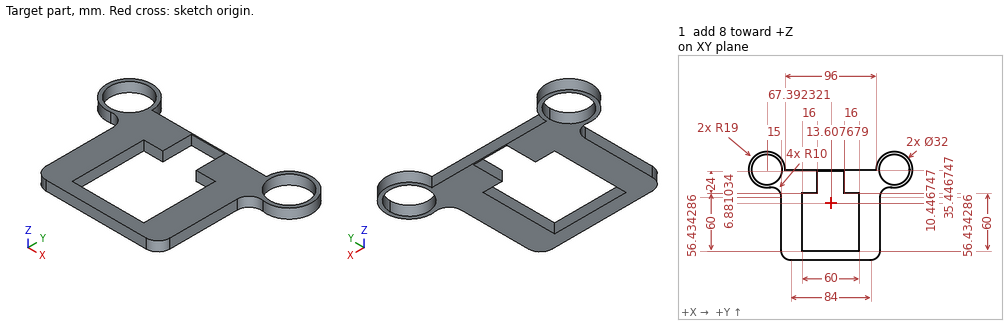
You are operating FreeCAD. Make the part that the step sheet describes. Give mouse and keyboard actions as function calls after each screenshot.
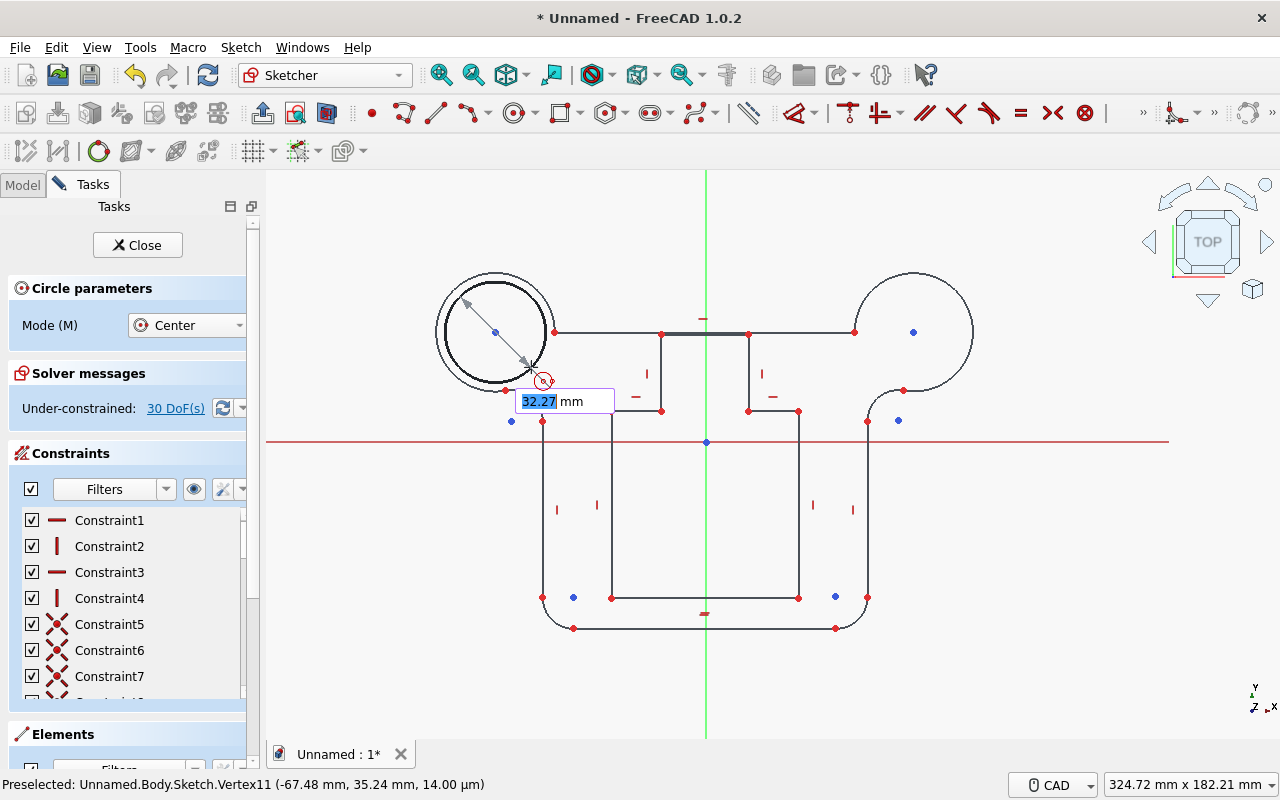
text(32)
key(Return)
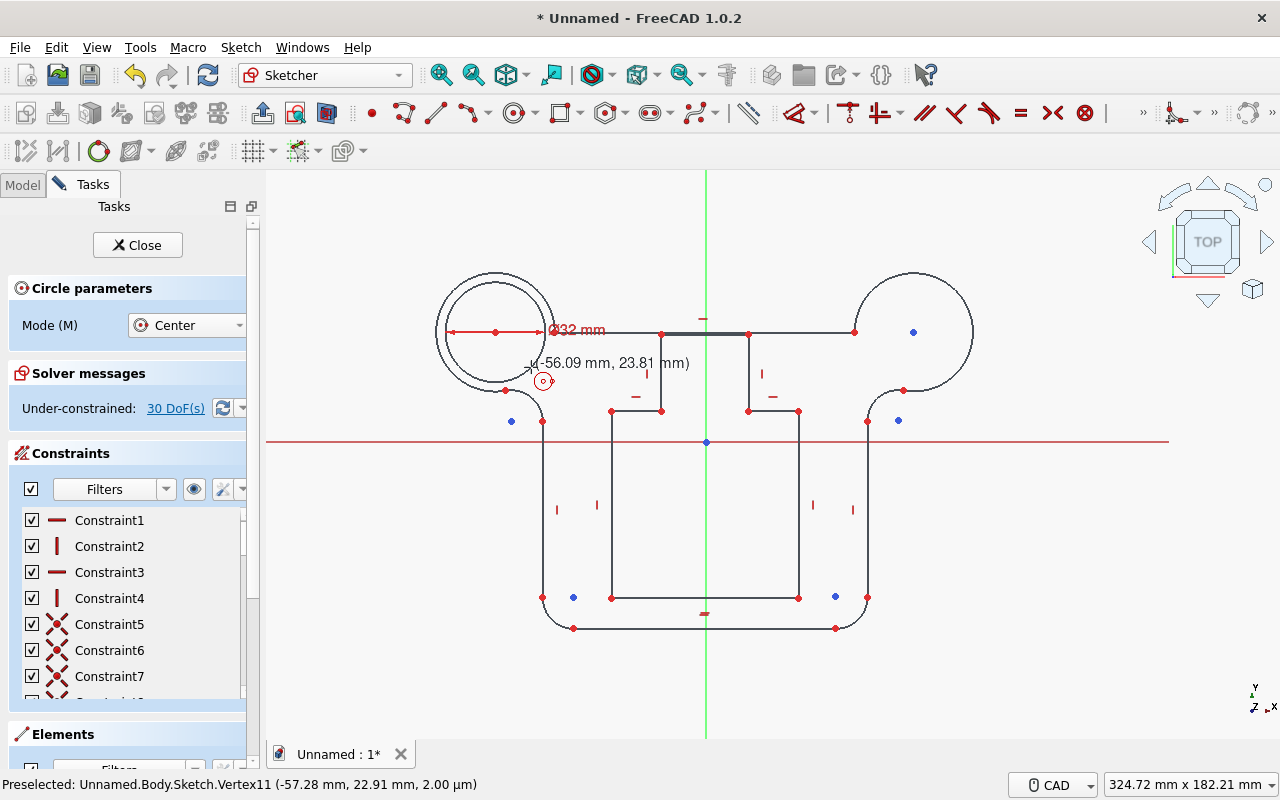
click(914, 332)
move(879, 367)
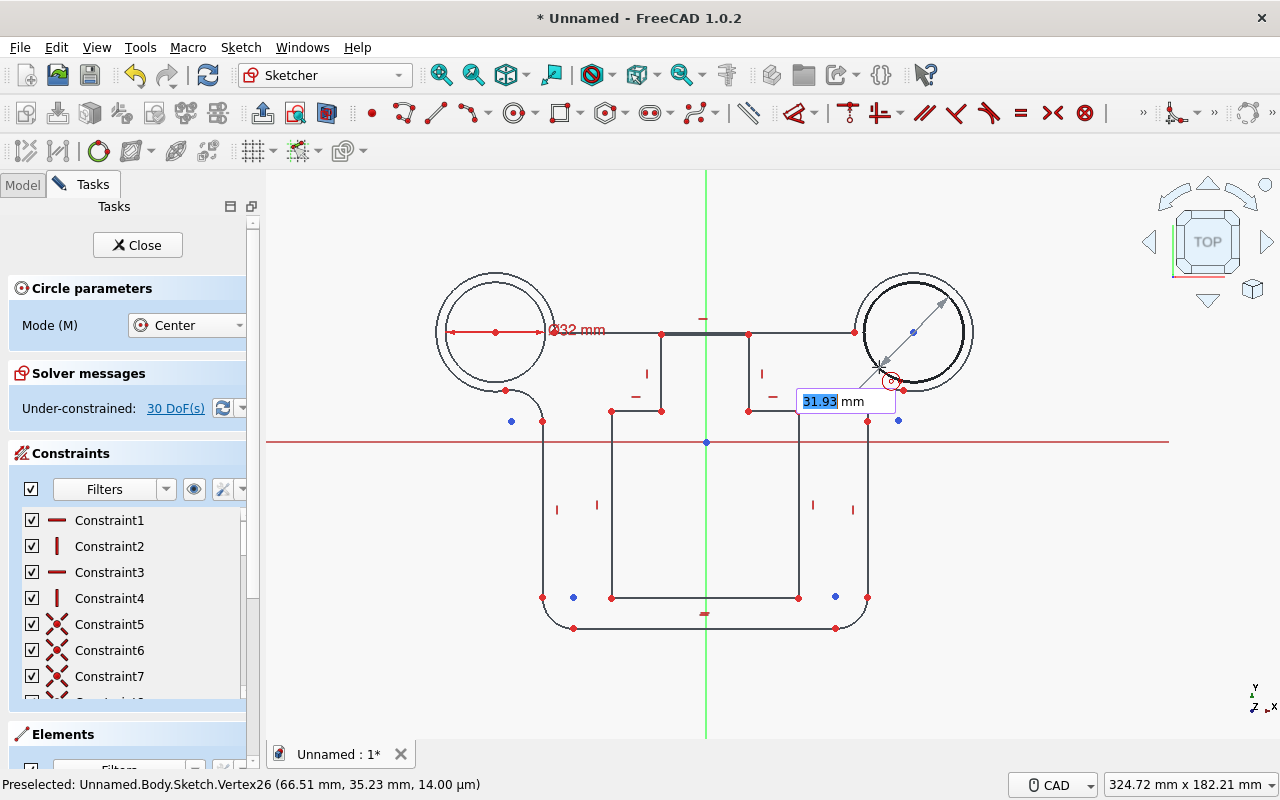
text(32)
key(Return)
key(Escape)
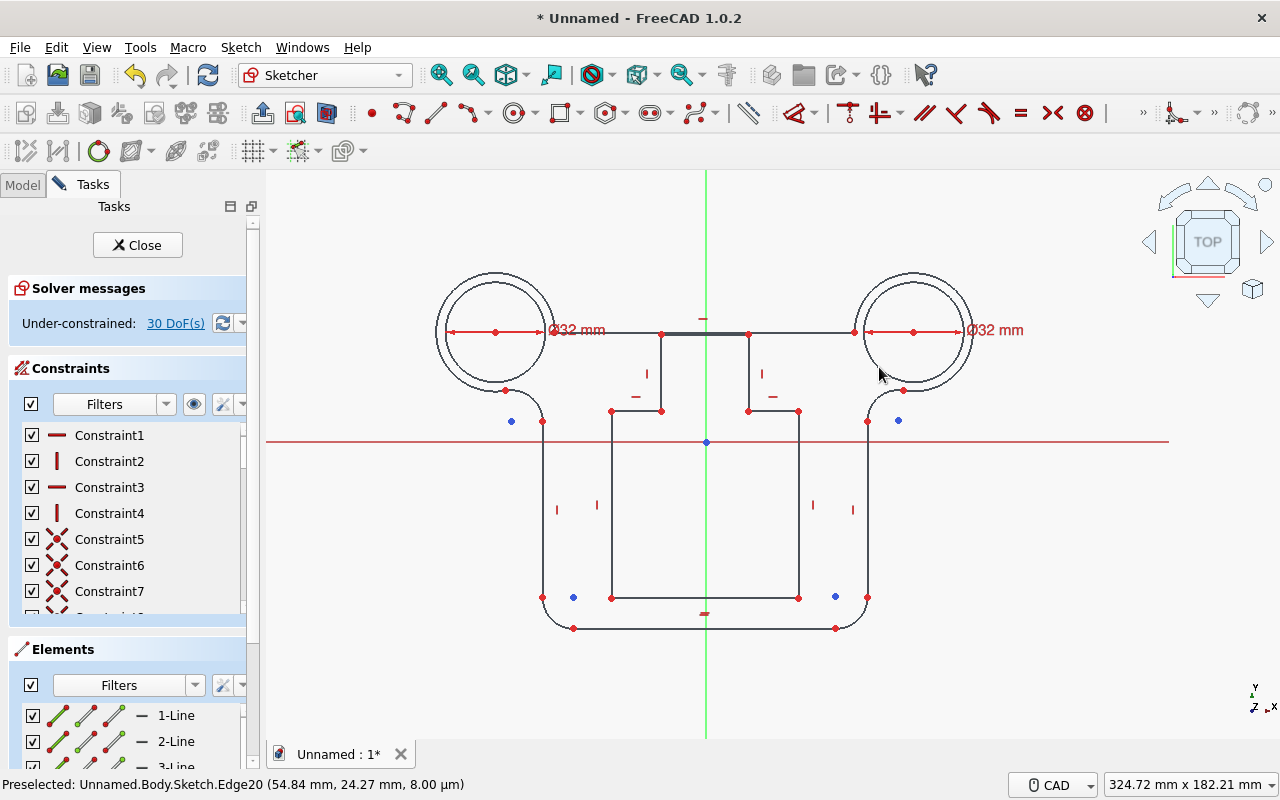
click(543, 474)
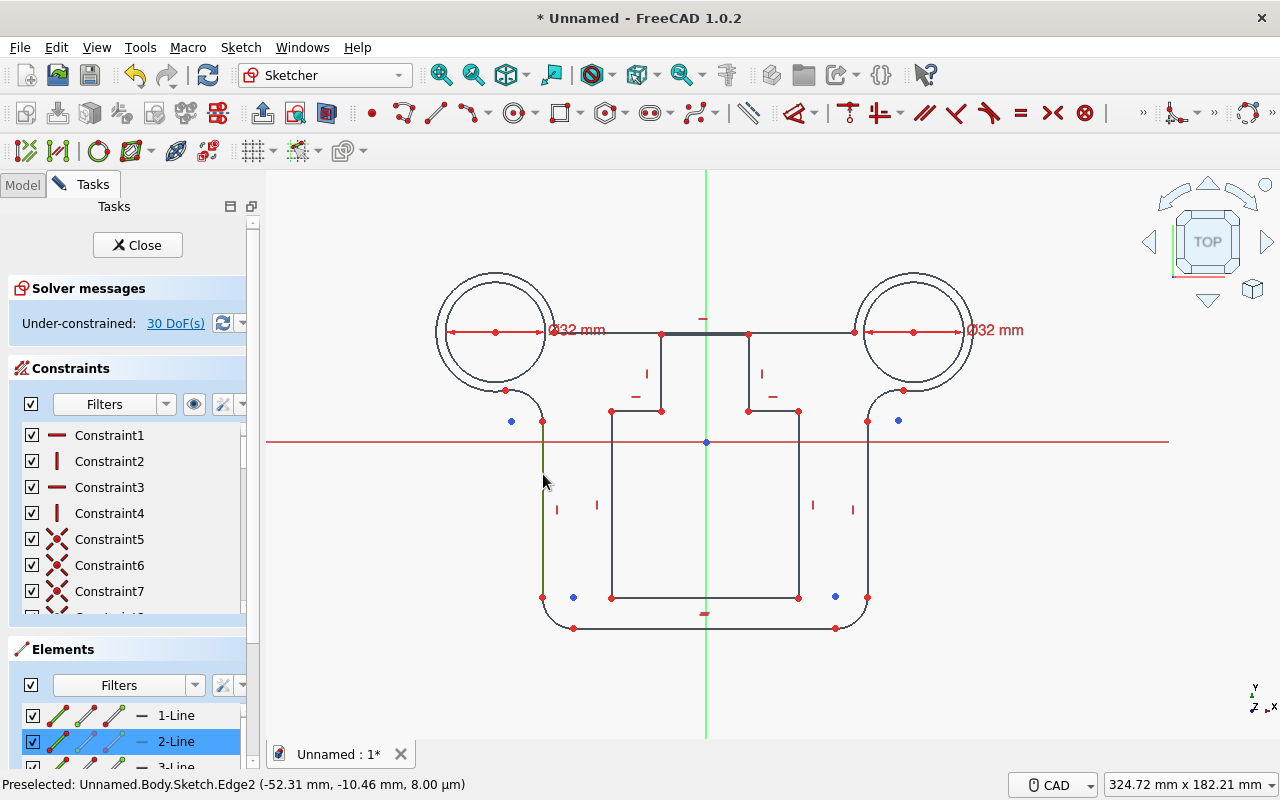
click(538, 406)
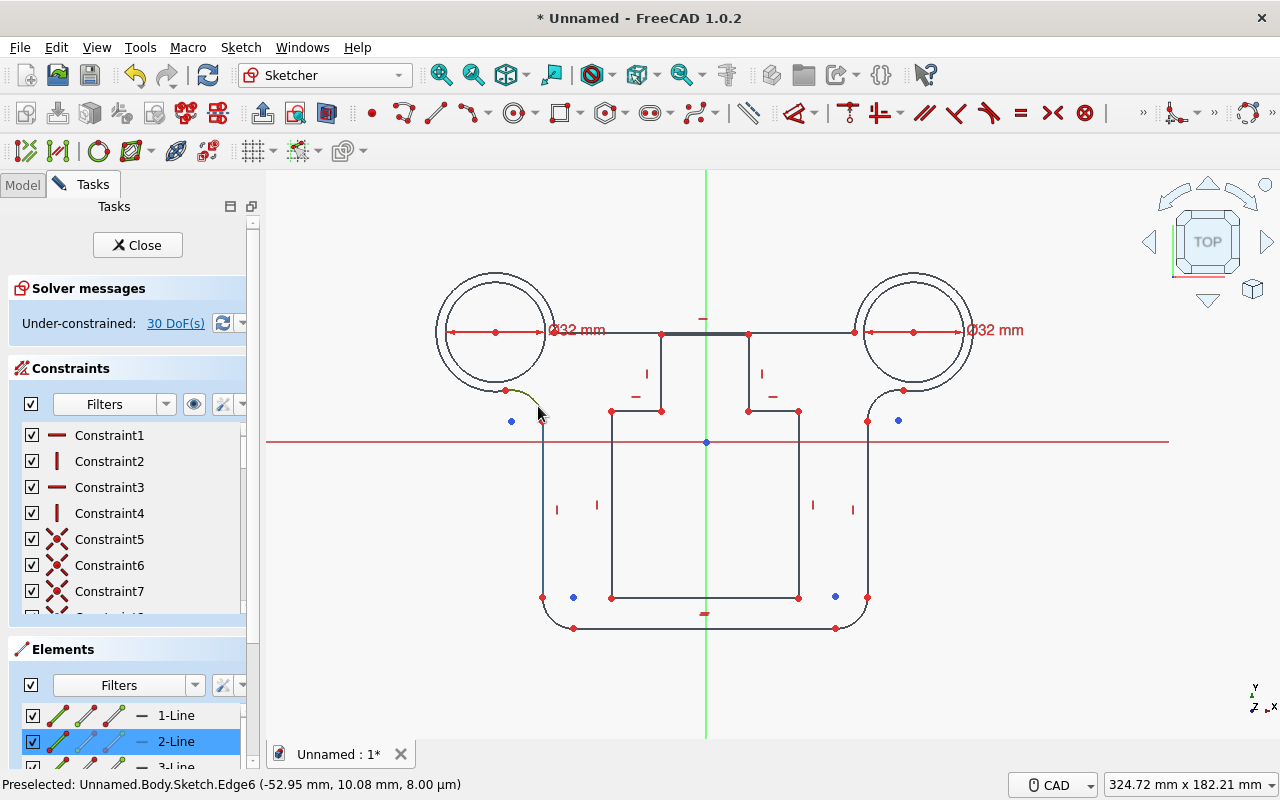
click(990, 114)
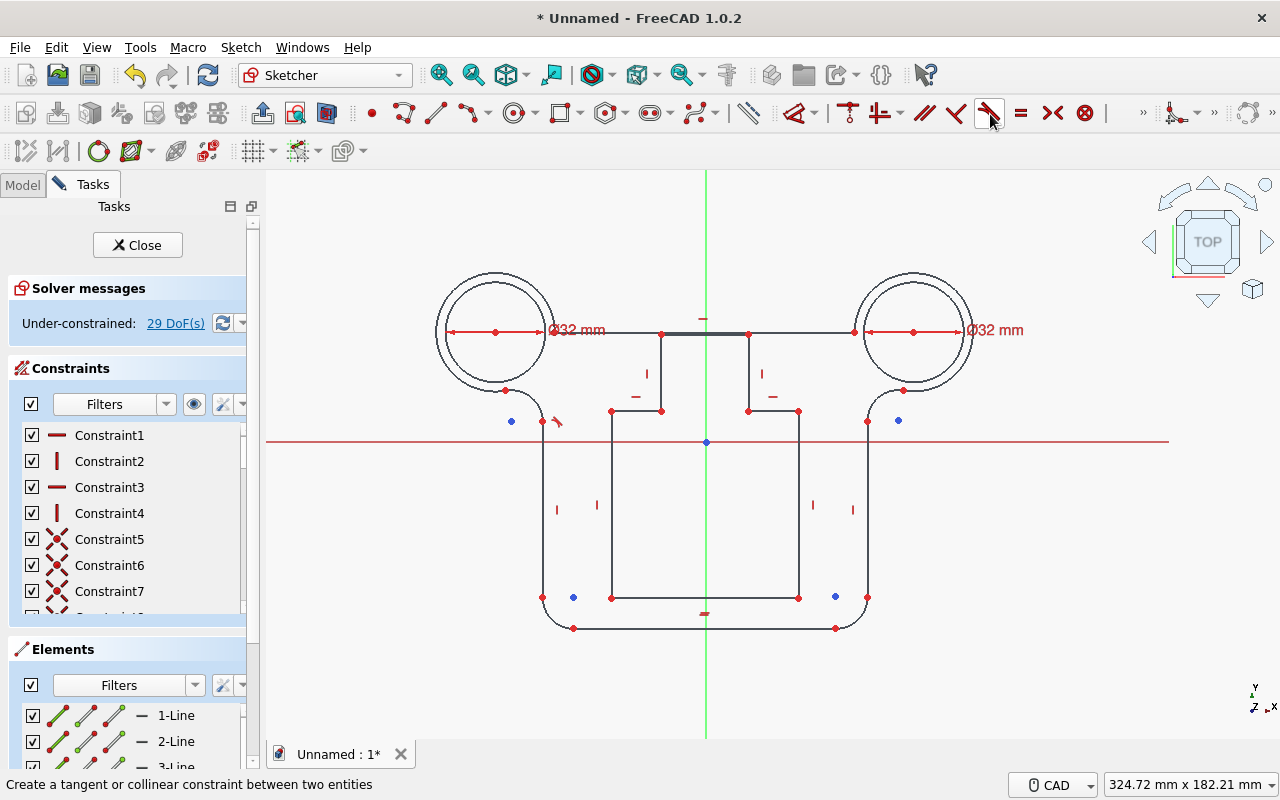
click(543, 475)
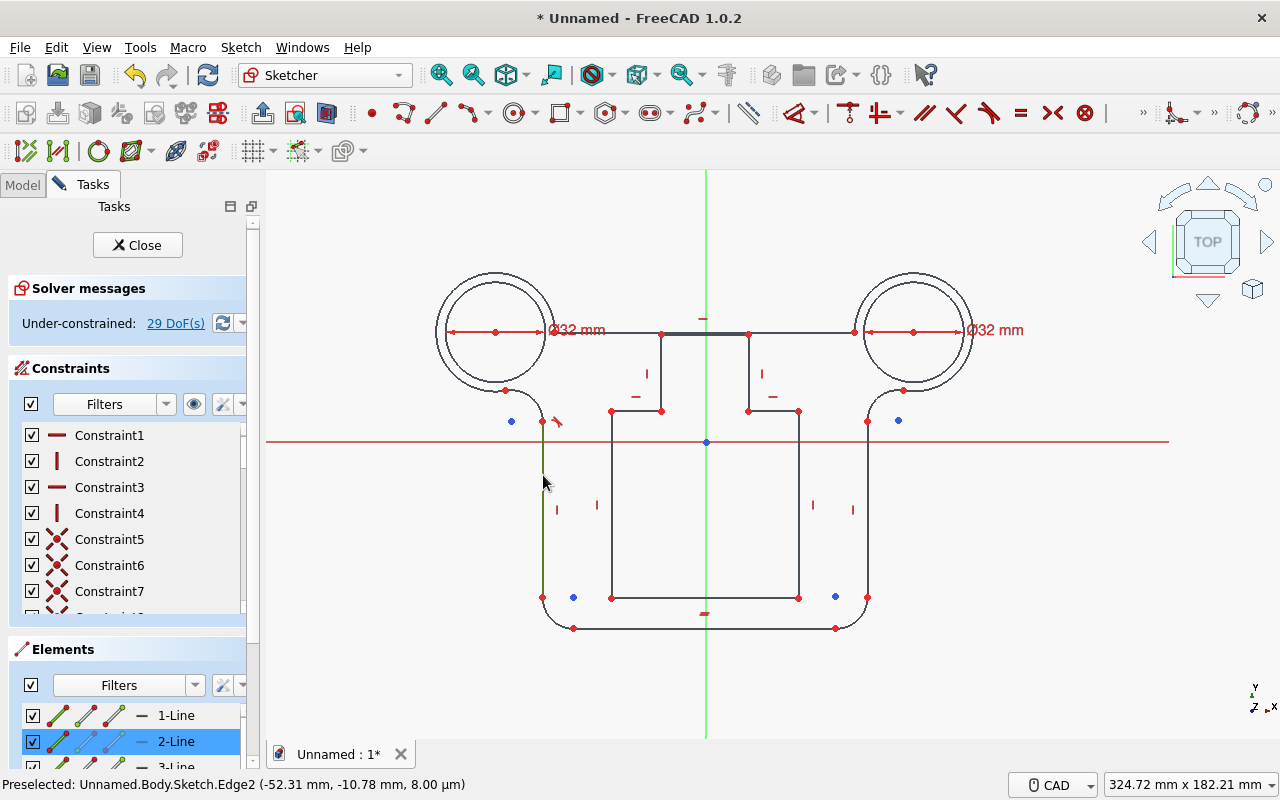
click(546, 612)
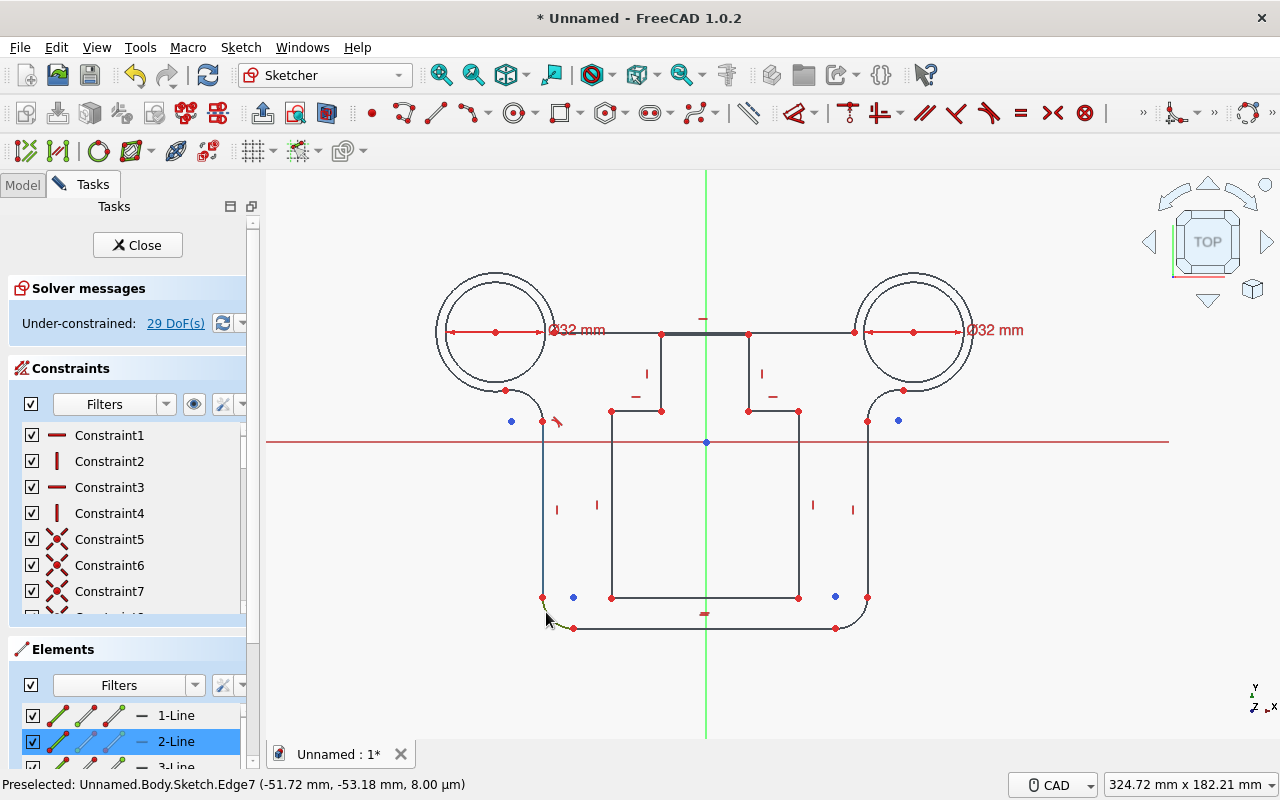
click(990, 114)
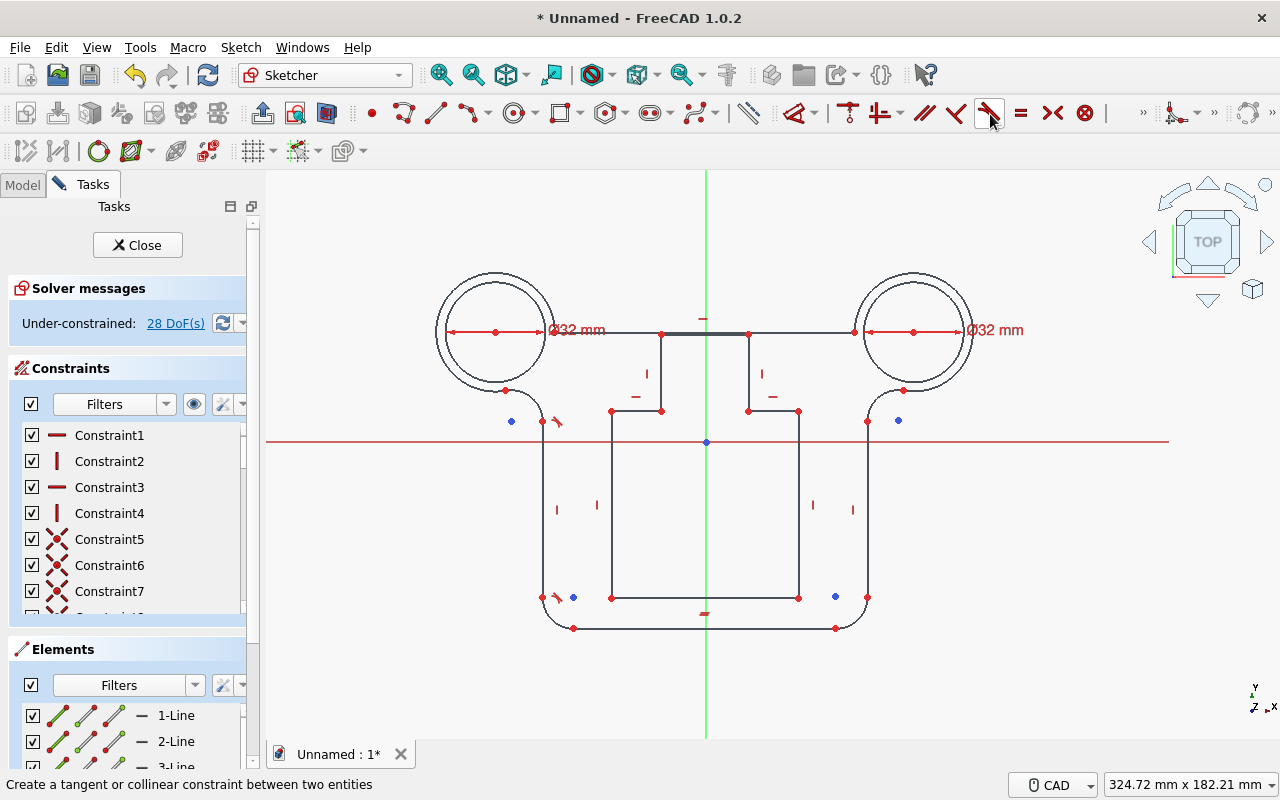
click(652, 629)